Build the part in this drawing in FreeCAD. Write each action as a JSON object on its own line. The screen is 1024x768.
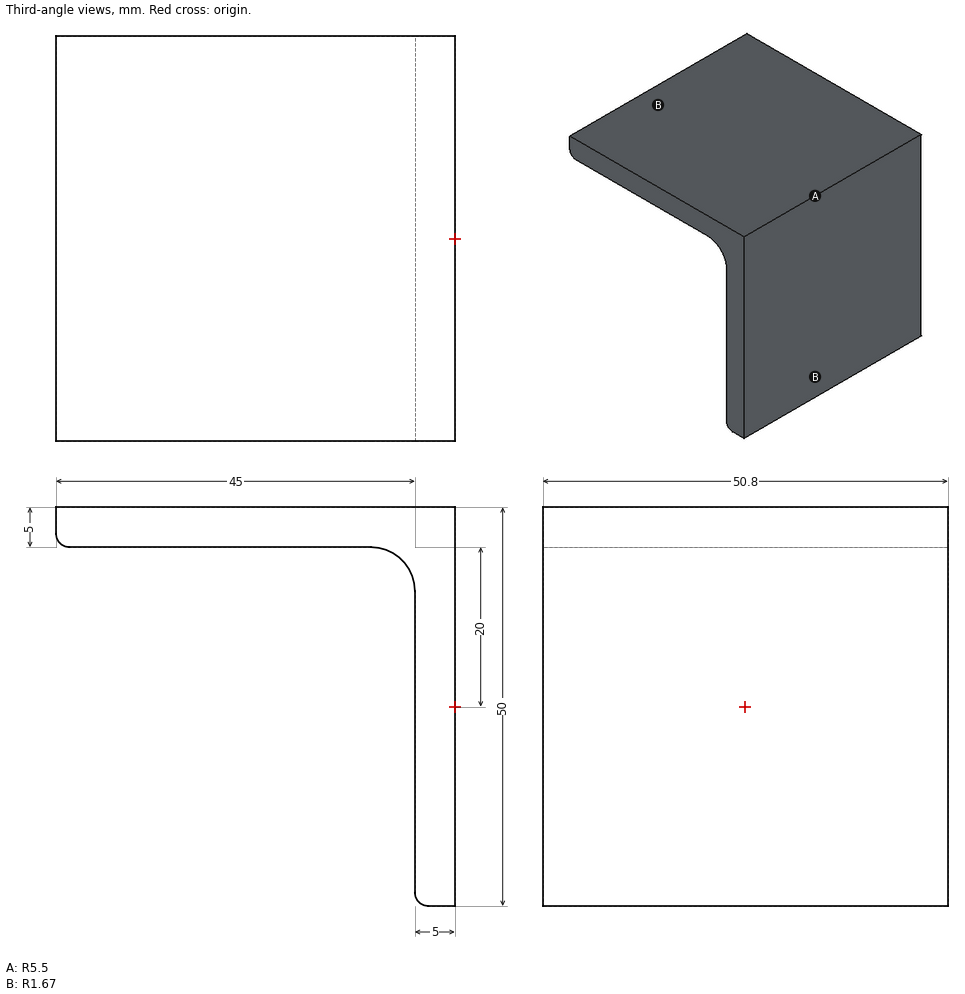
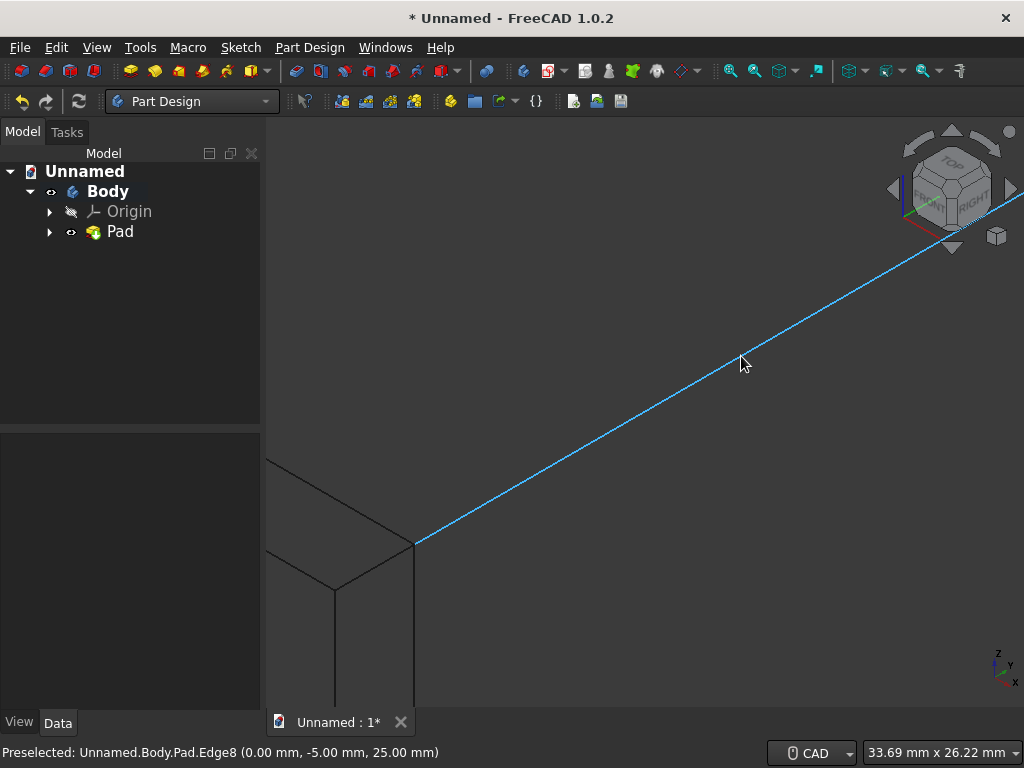
{"action": "left_click", "coordinate": [732, 72]}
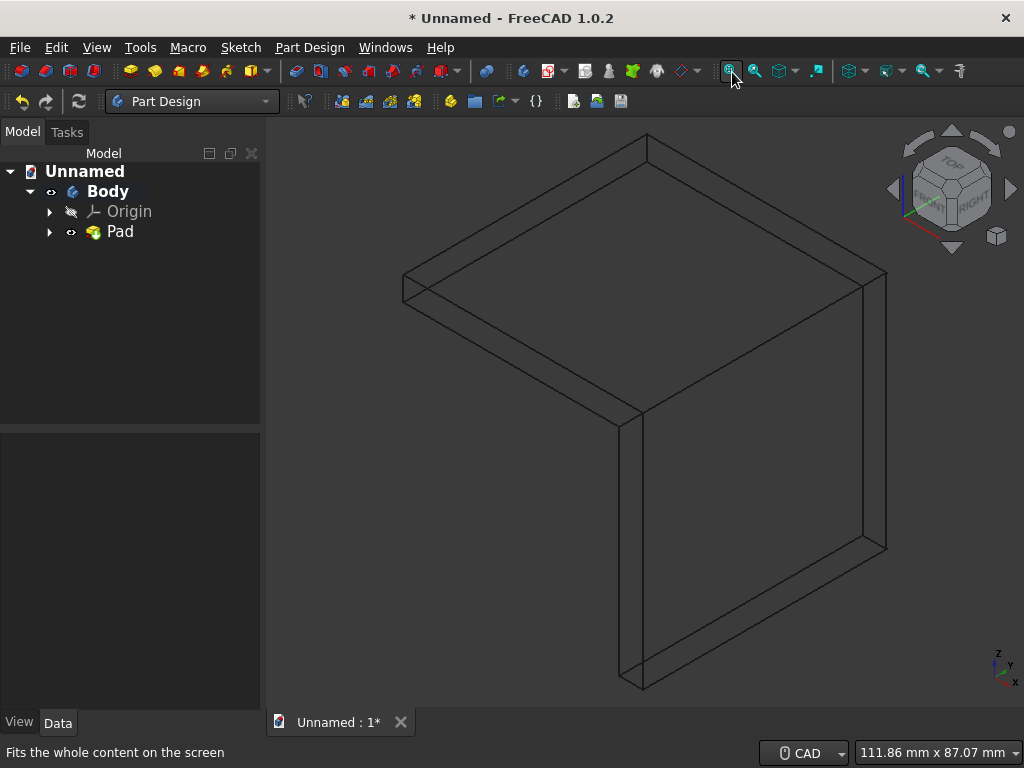
{"action": "key", "text": "2"}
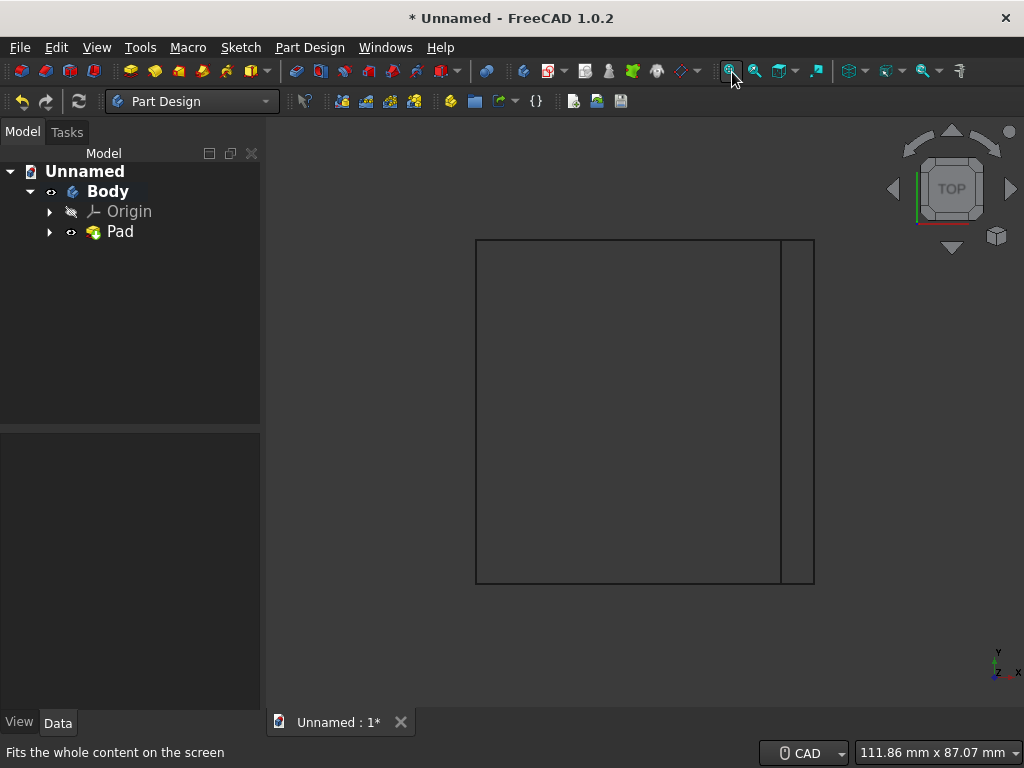
{"action": "left_click", "coordinate": [781, 411]}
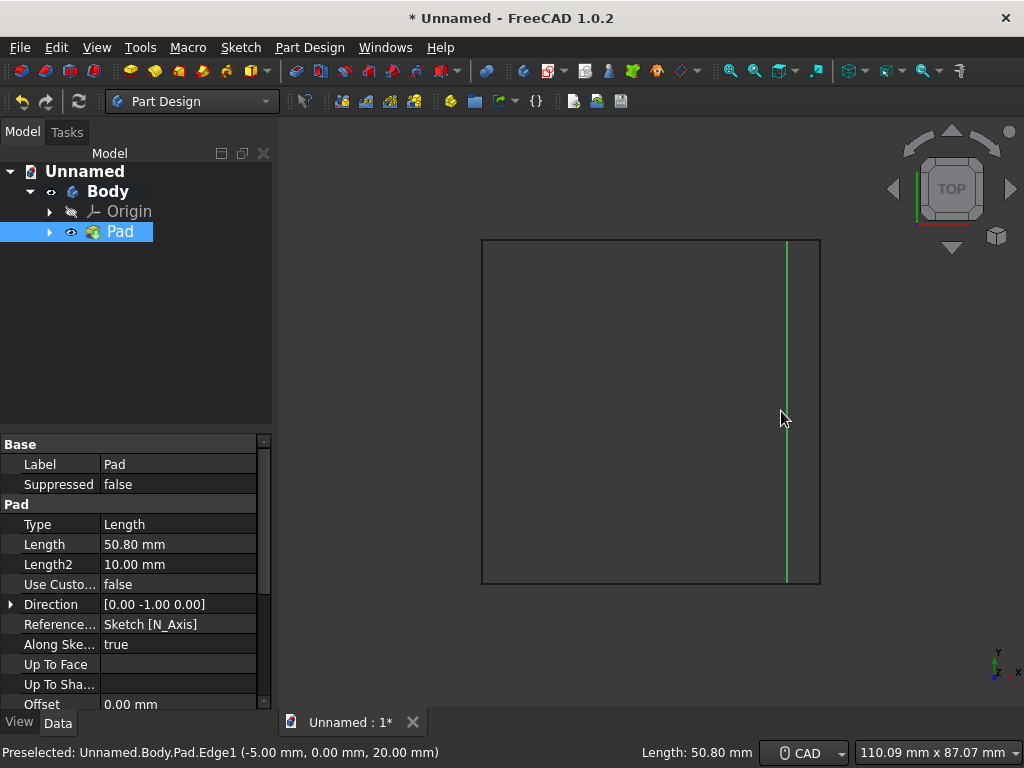
{"action": "key", "text": "v 1"}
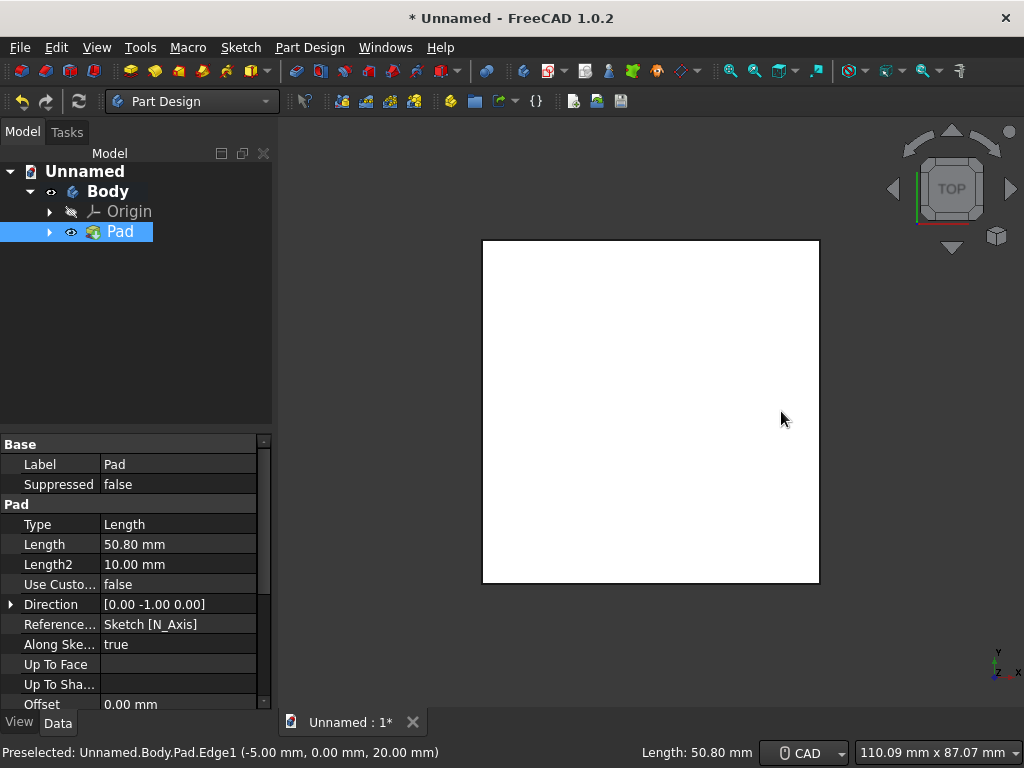
{"action": "left_click", "coordinate": [22, 72]}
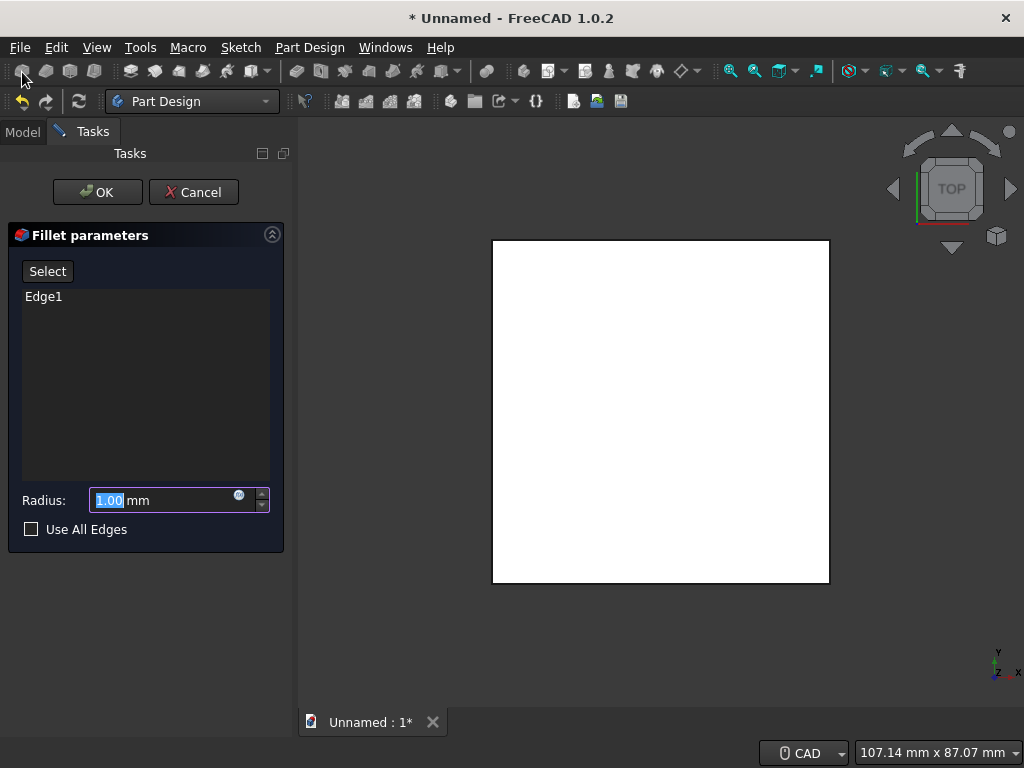
{"action": "type", "text": "5.5"}
{"action": "key", "text": "Tab"}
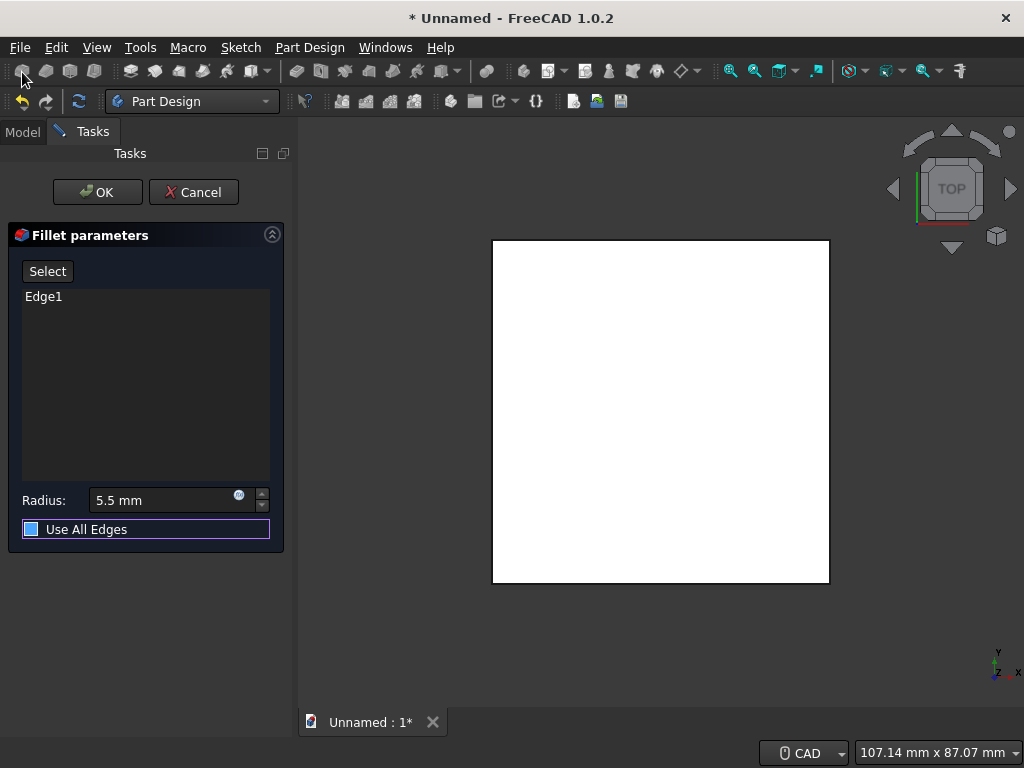
{"action": "left_click", "coordinate": [98, 192]}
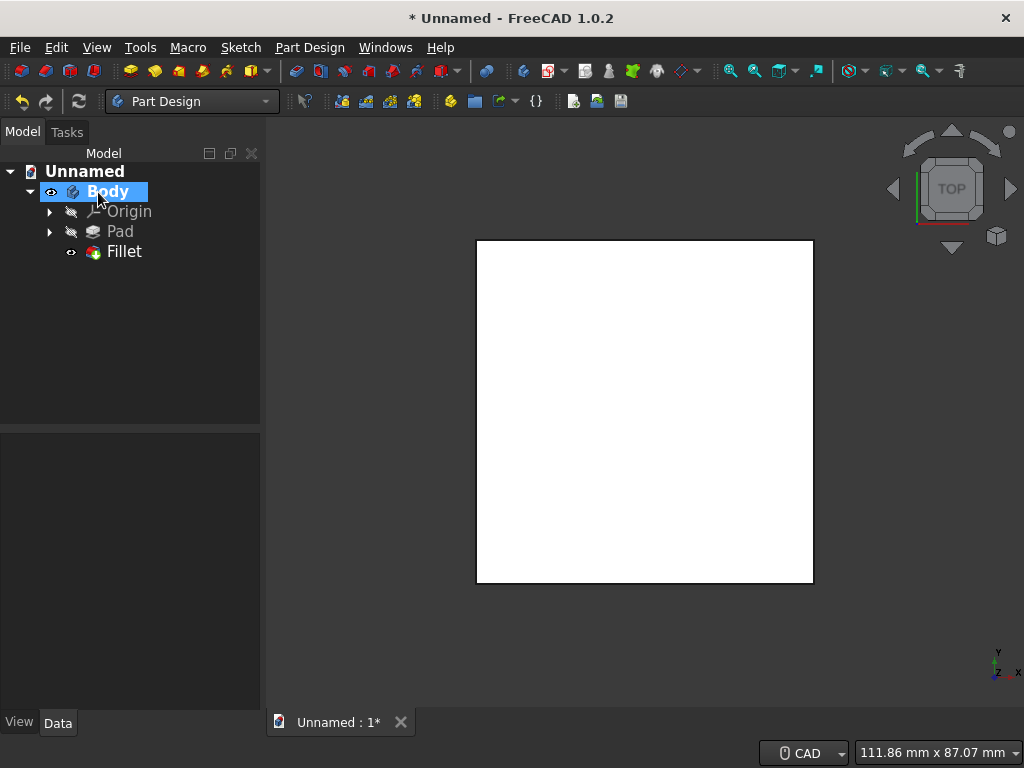
{"action": "key", "text": "0"}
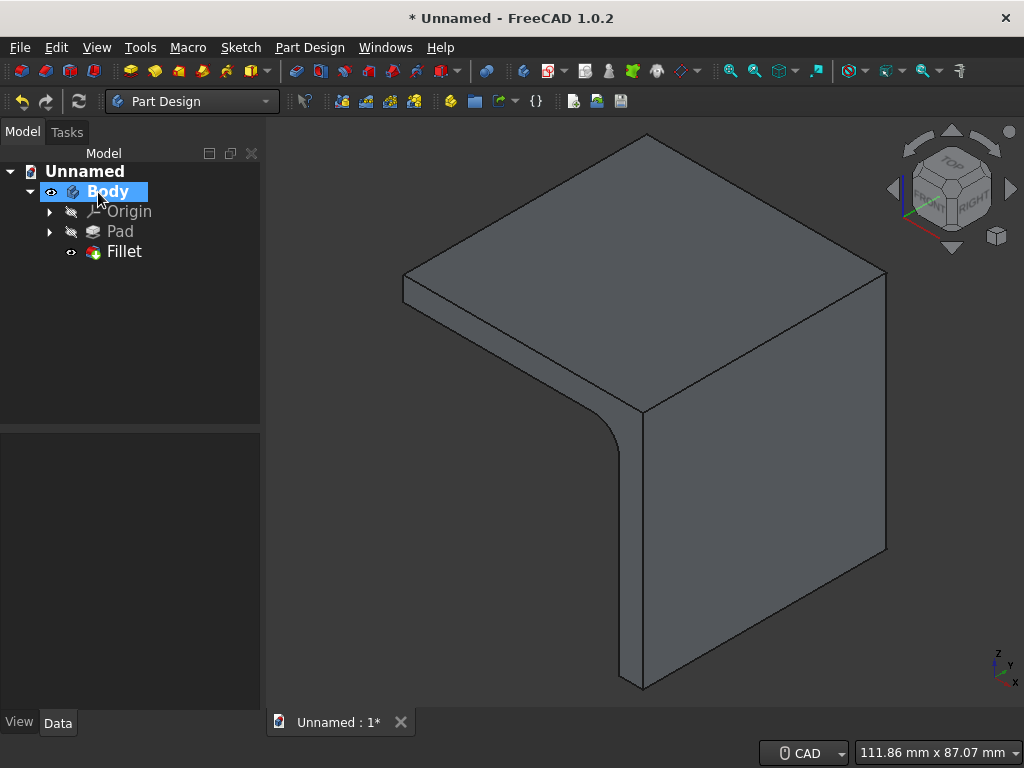
{"action": "key", "text": "2"}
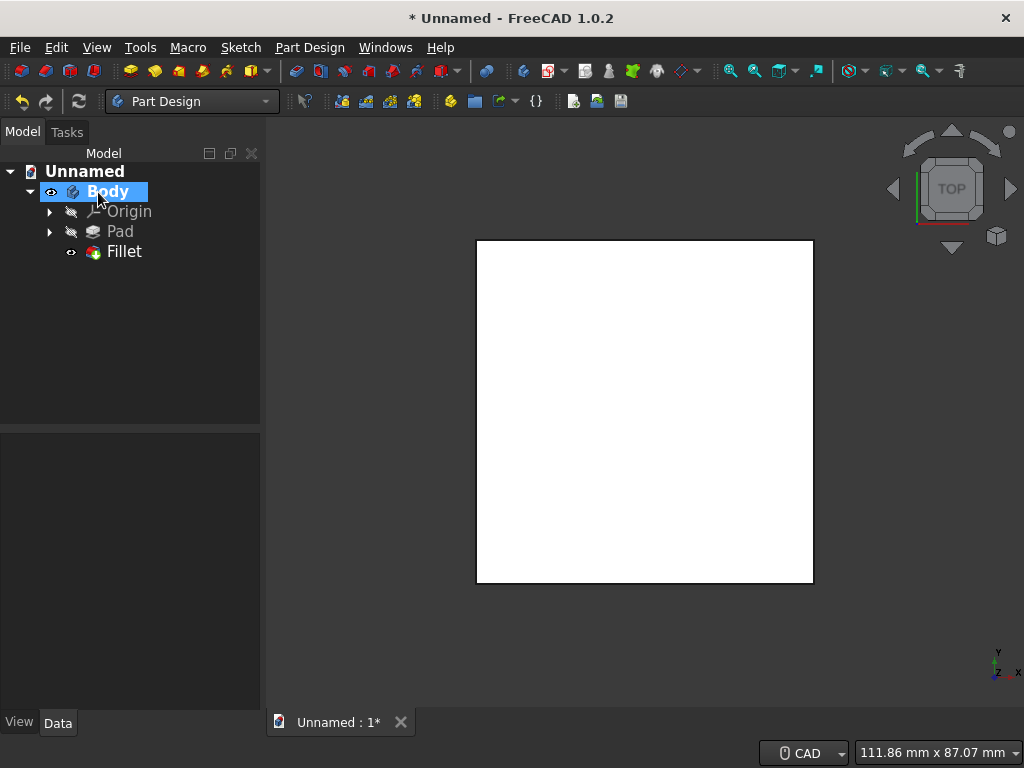
{"action": "key", "text": "1"}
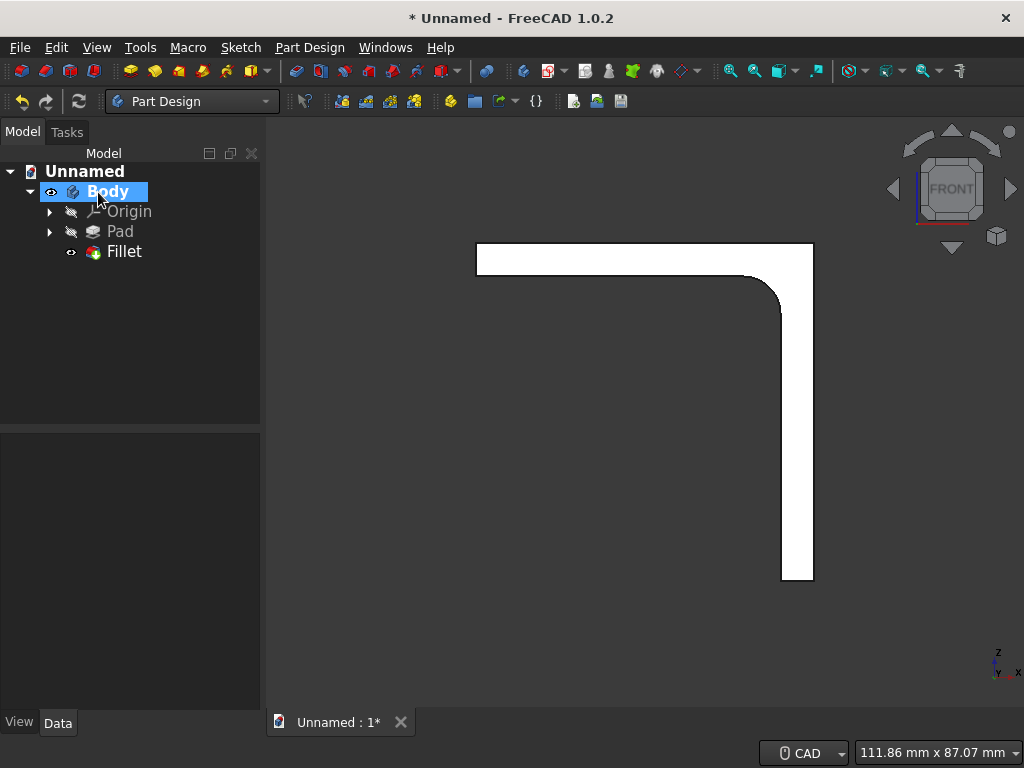
{"action": "key", "text": "3"}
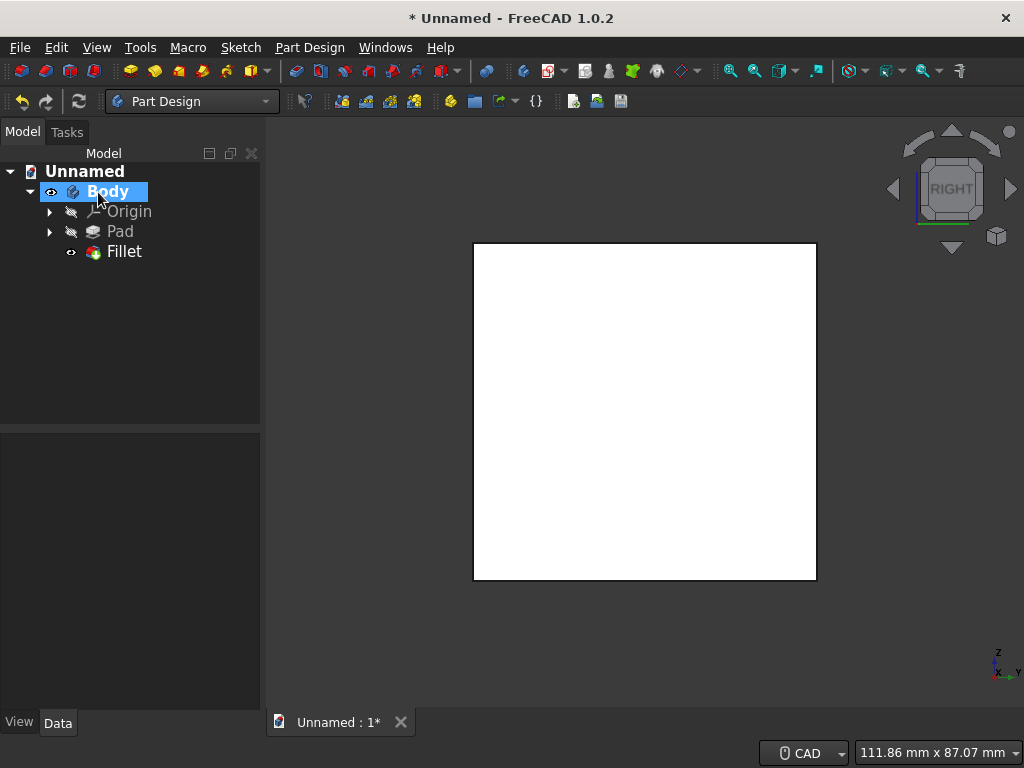
{"action": "key", "text": "5"}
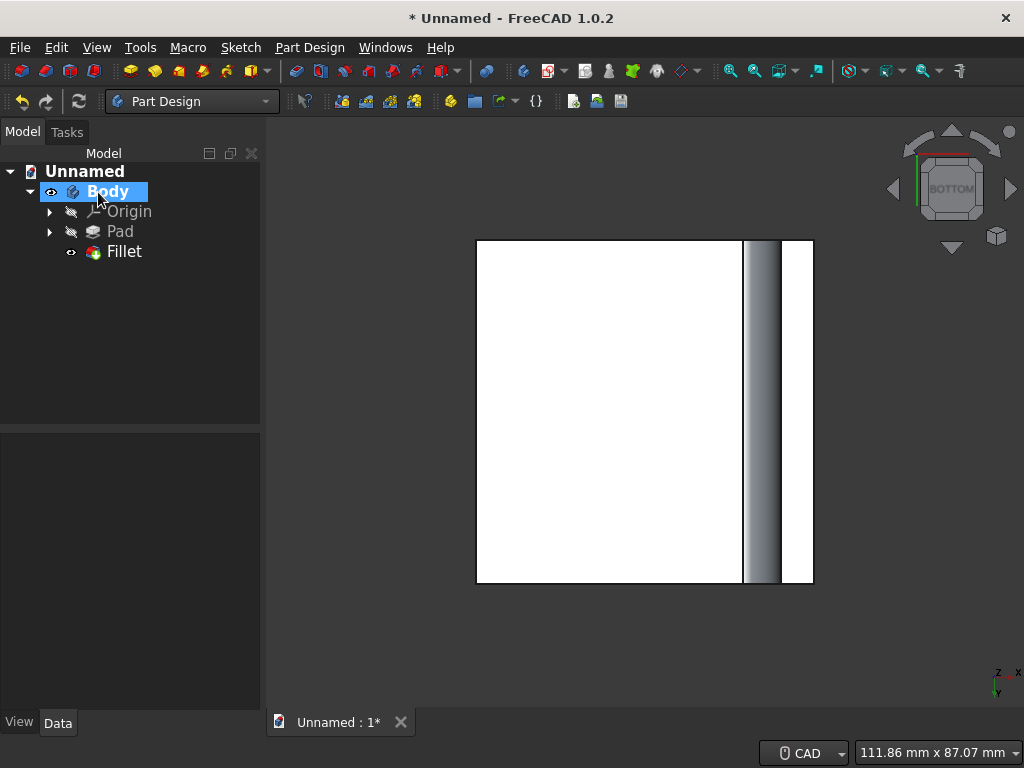
{"action": "left_click", "coordinate": [476, 411]}